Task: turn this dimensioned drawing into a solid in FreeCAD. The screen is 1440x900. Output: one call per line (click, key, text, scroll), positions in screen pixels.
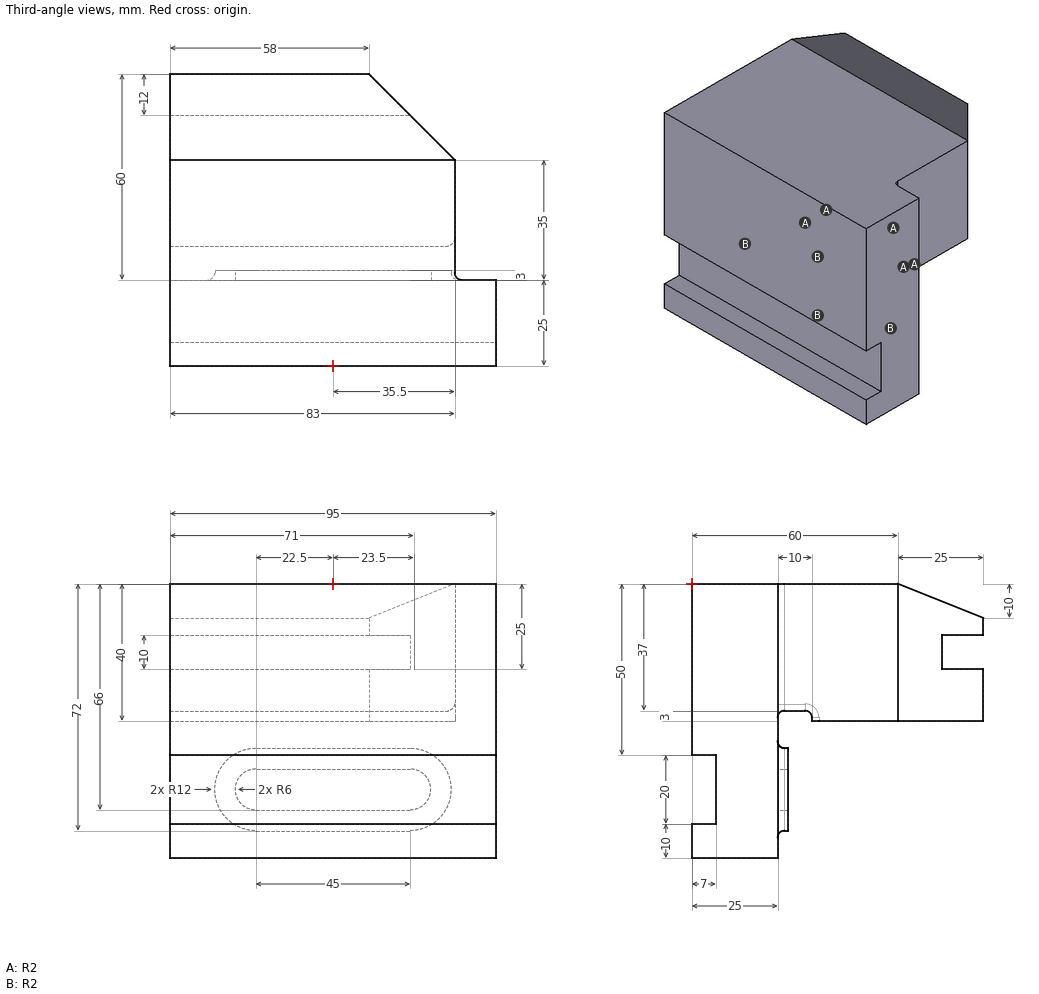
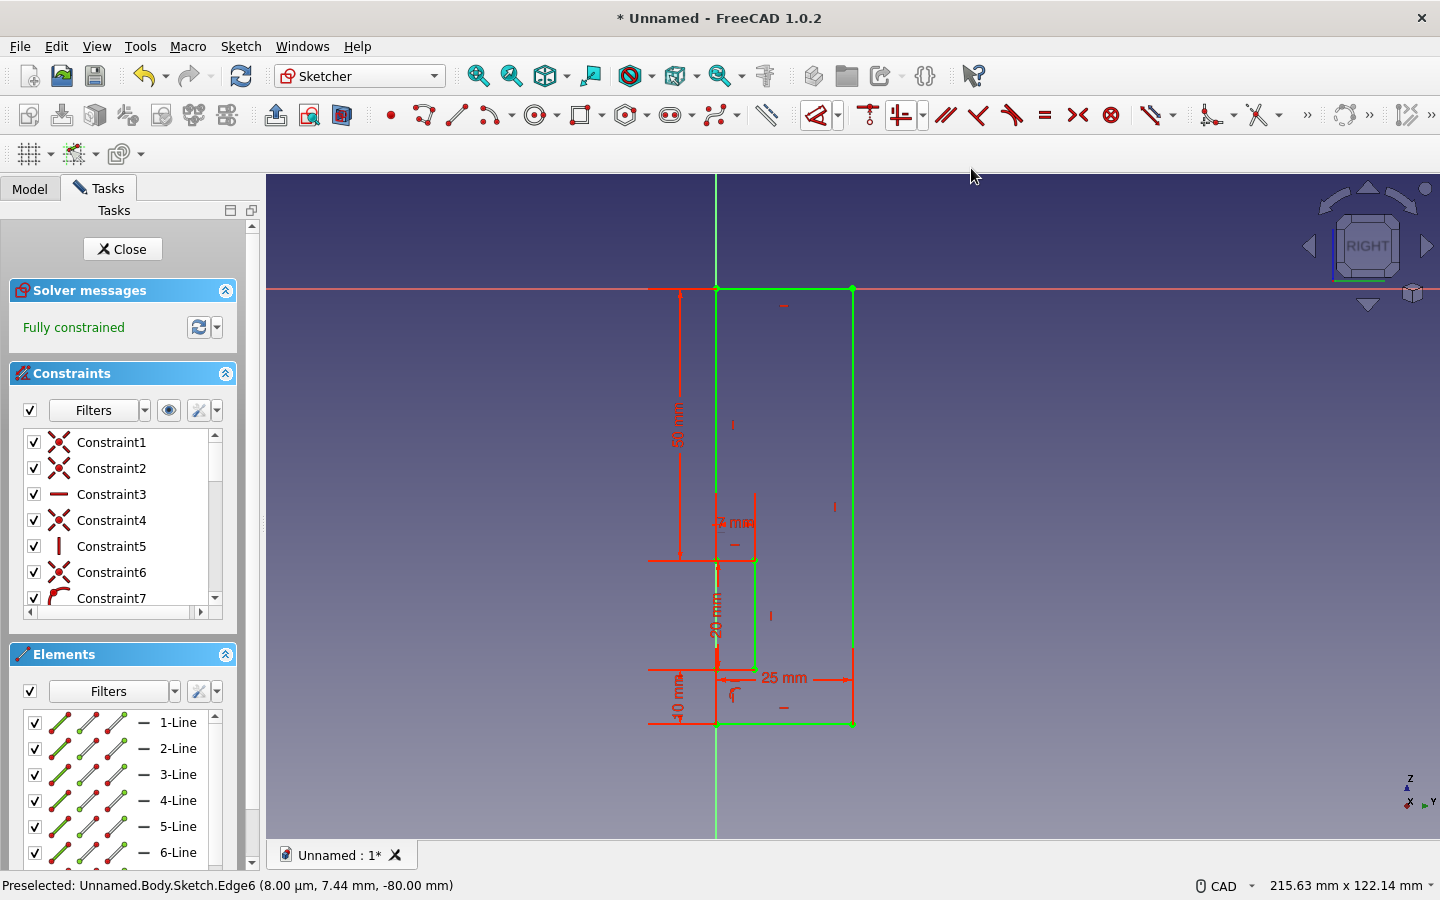
click(123, 249)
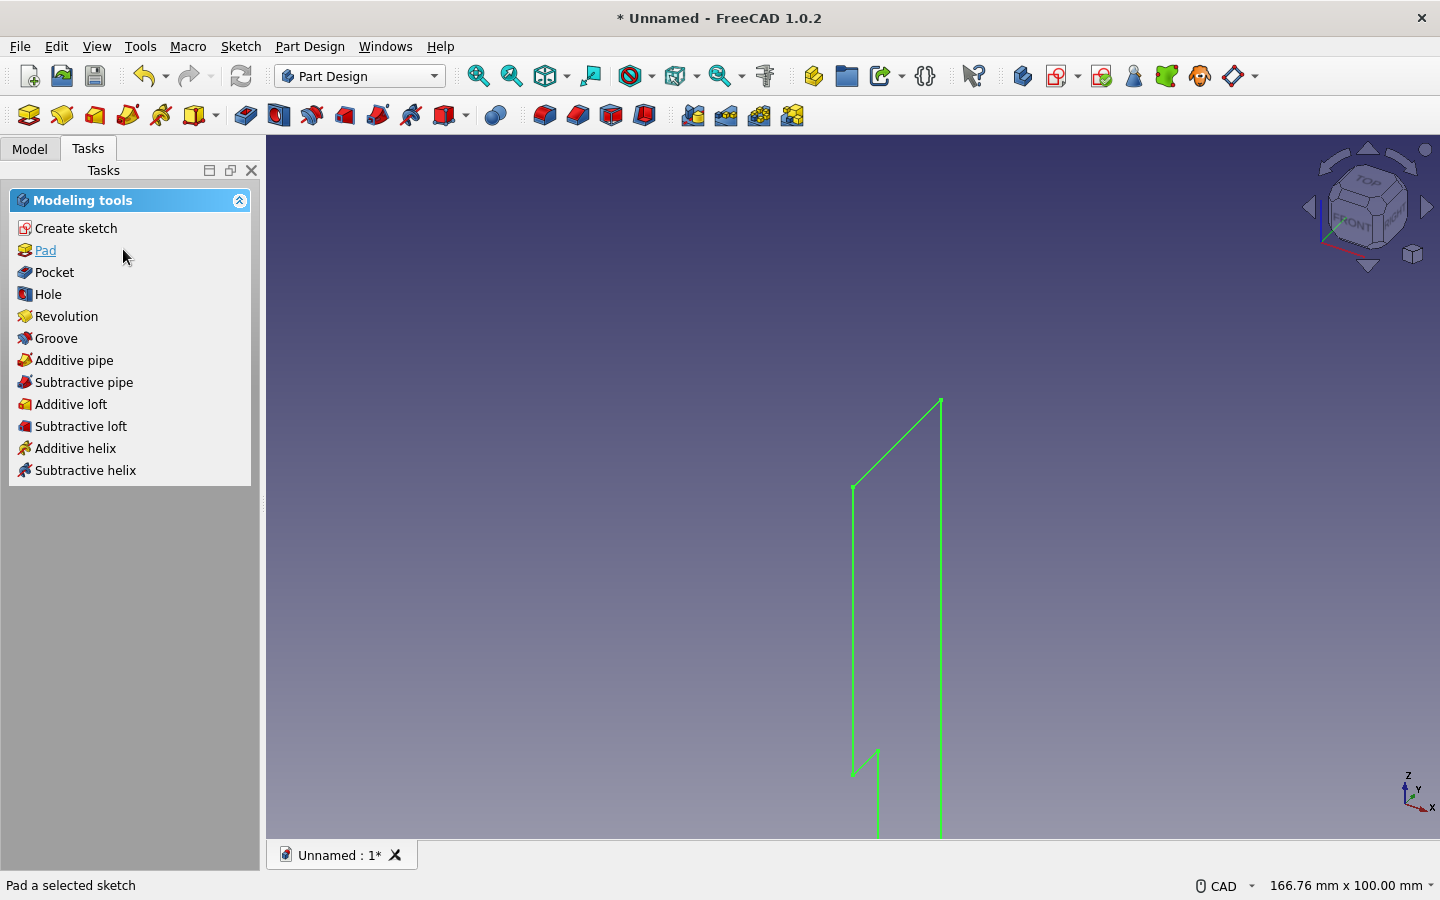
click(29, 116)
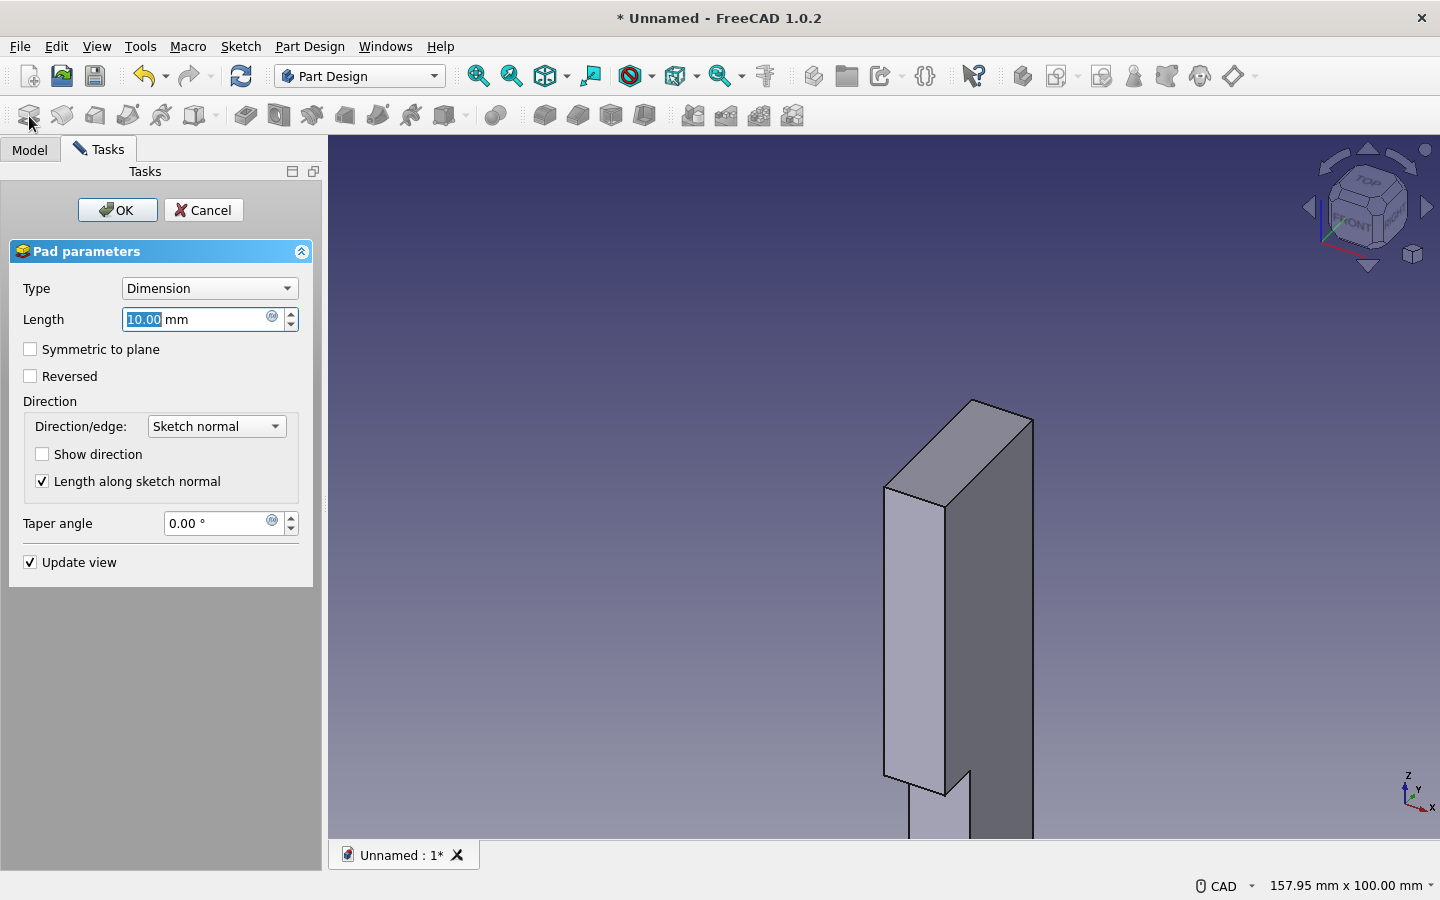
text(95)
key(Tab)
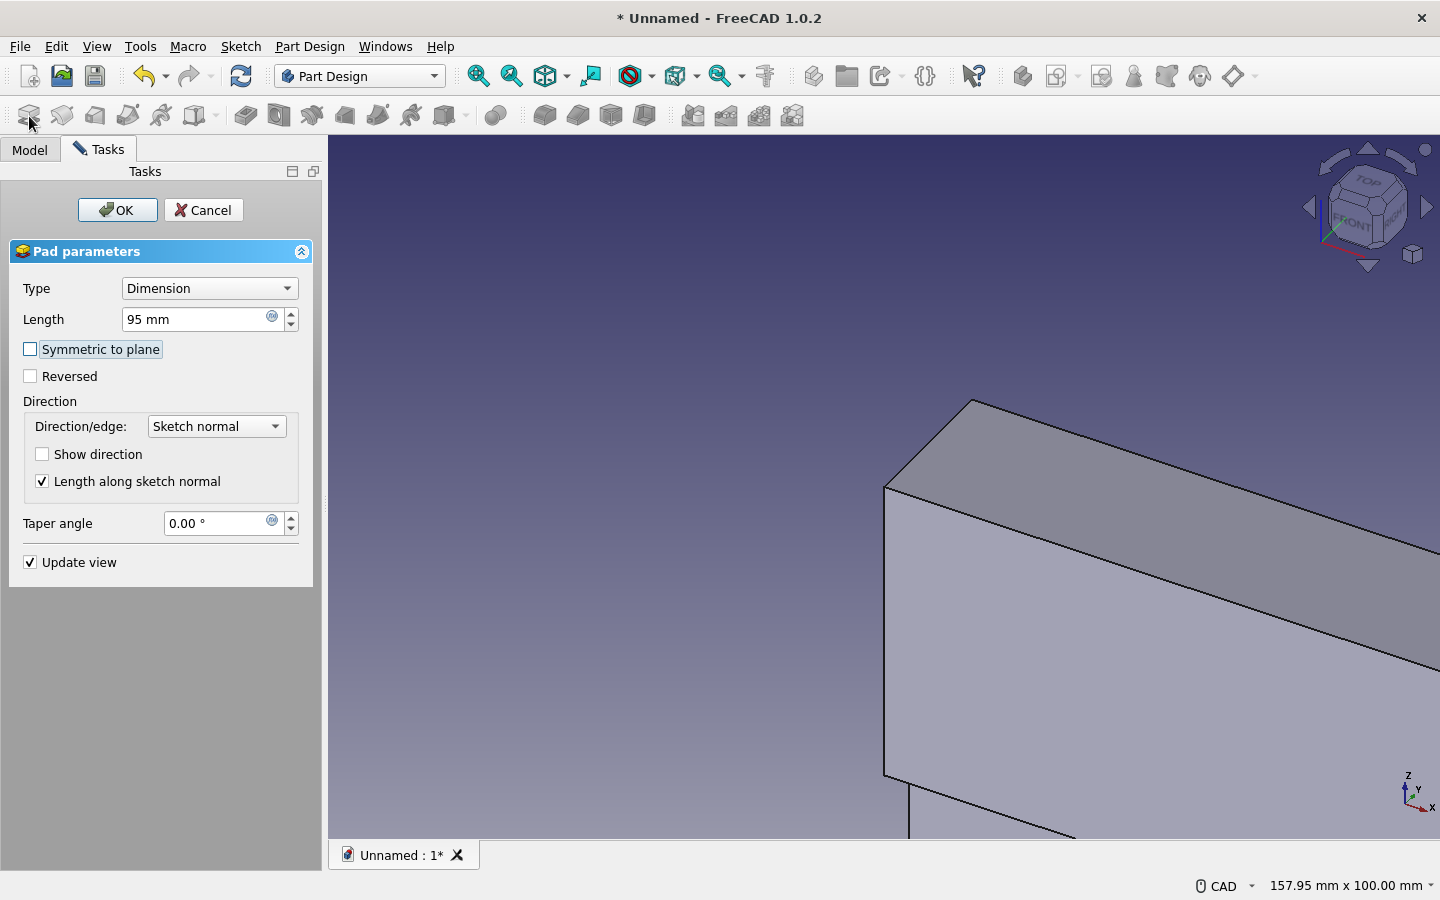
click(31, 349)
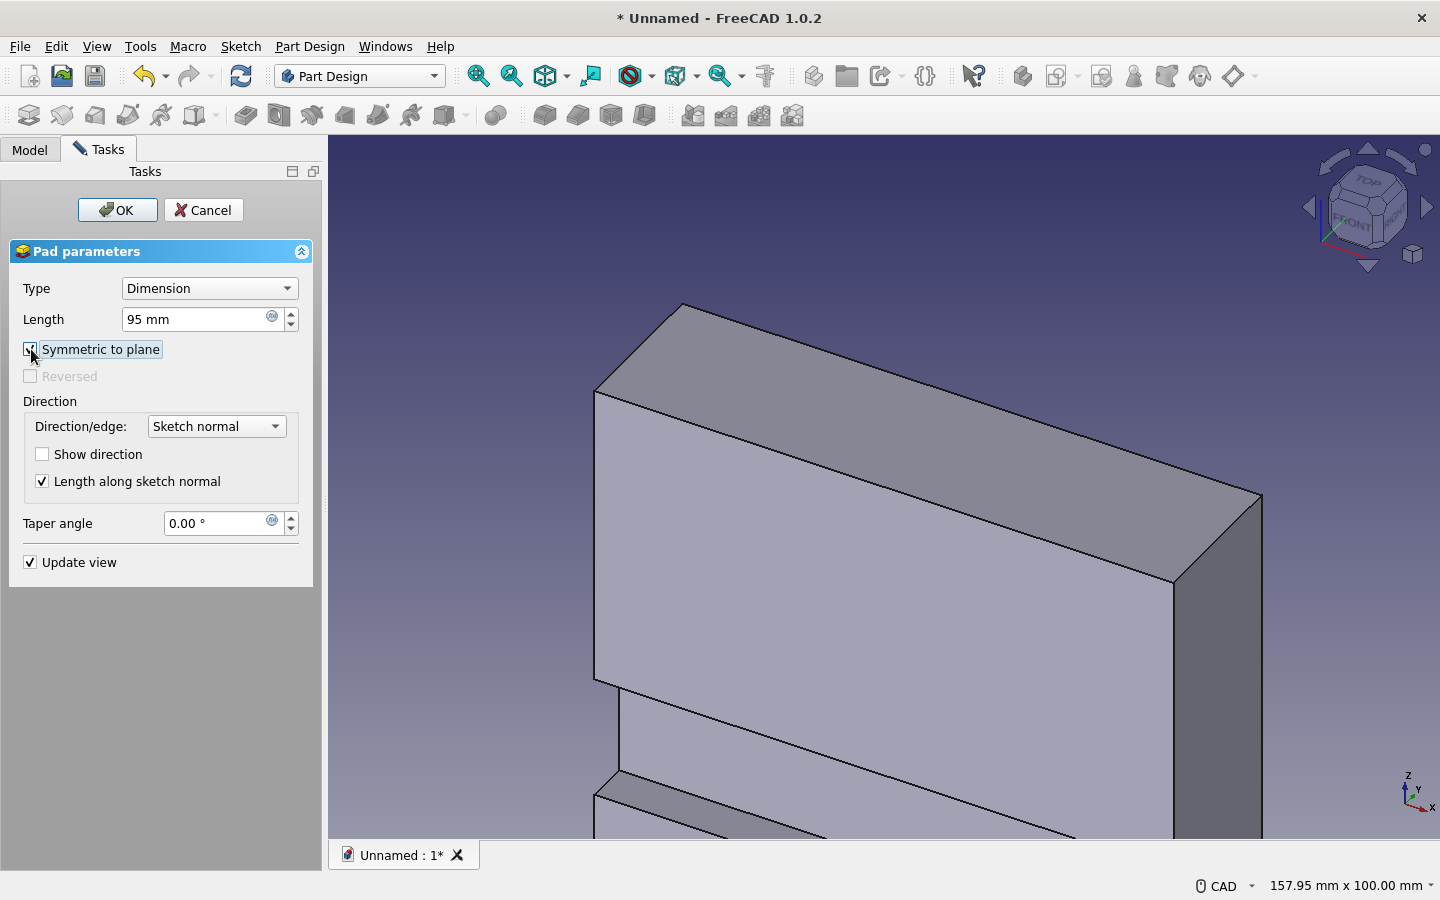
click(118, 210)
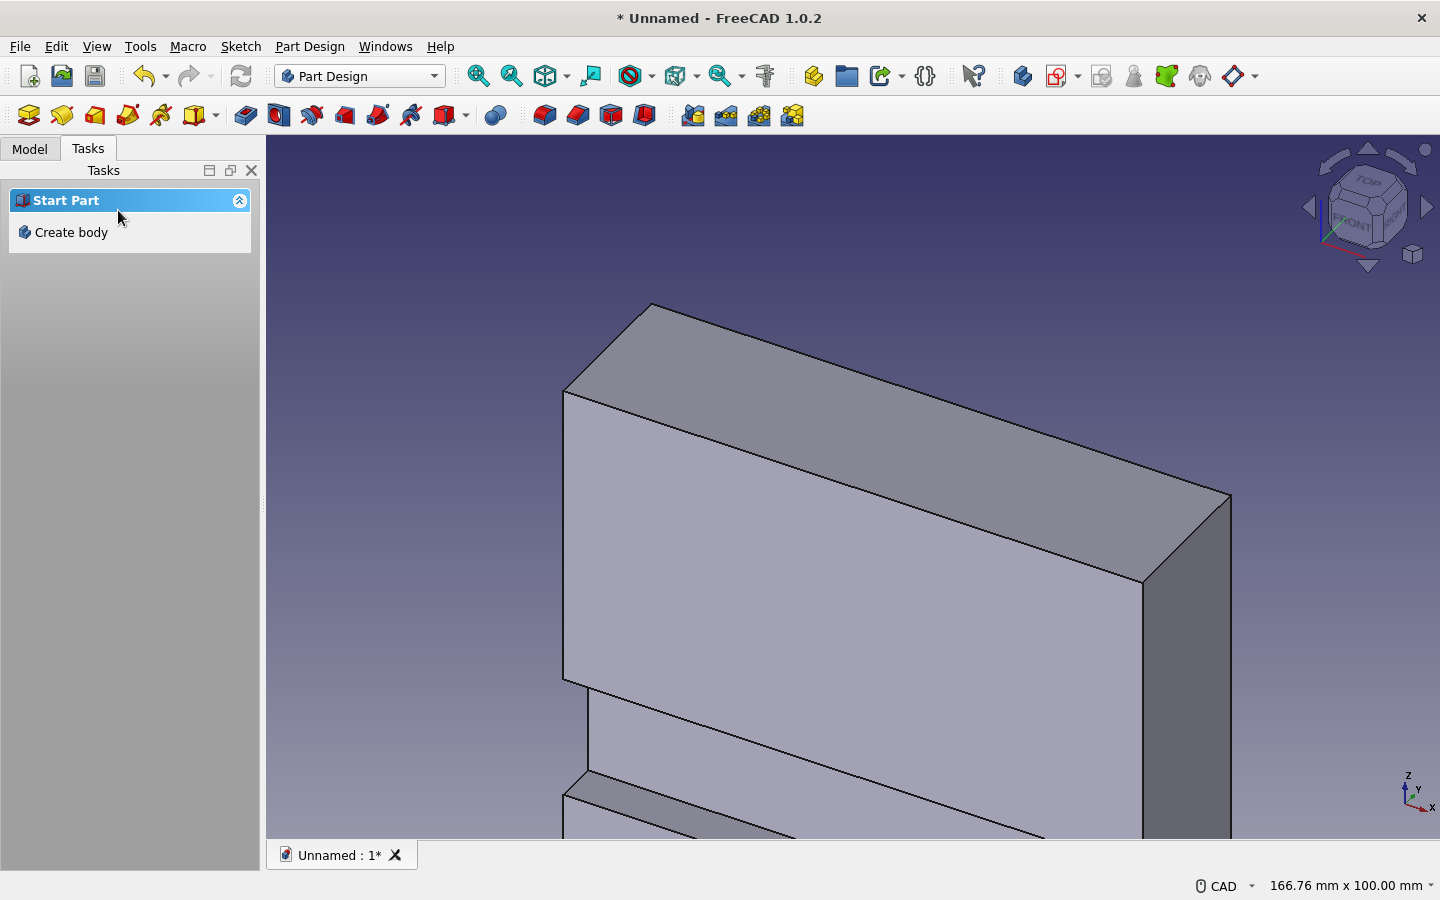
click(479, 76)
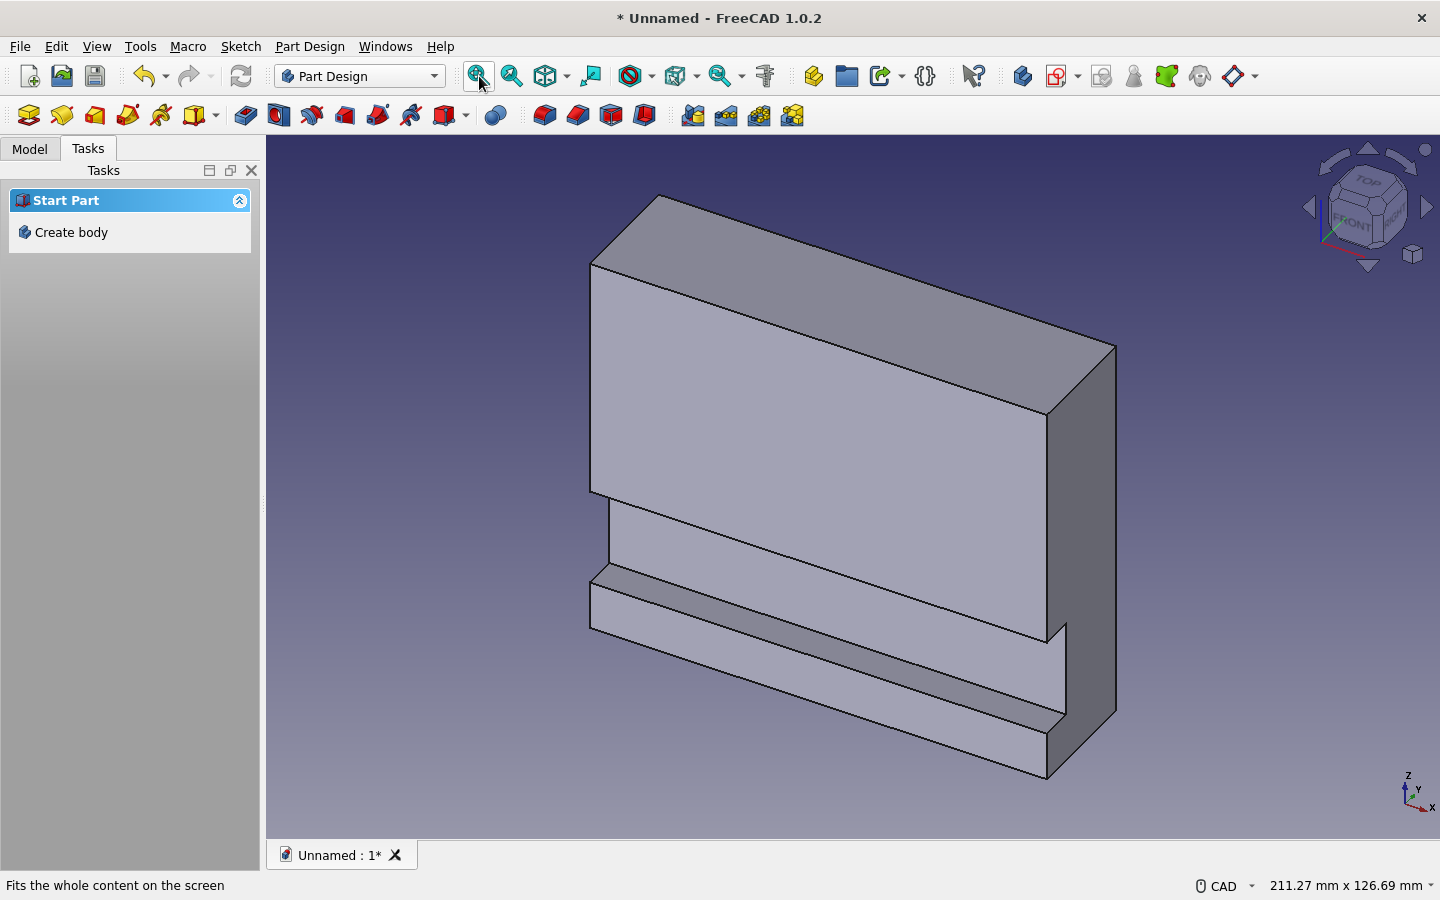
click(1056, 76)